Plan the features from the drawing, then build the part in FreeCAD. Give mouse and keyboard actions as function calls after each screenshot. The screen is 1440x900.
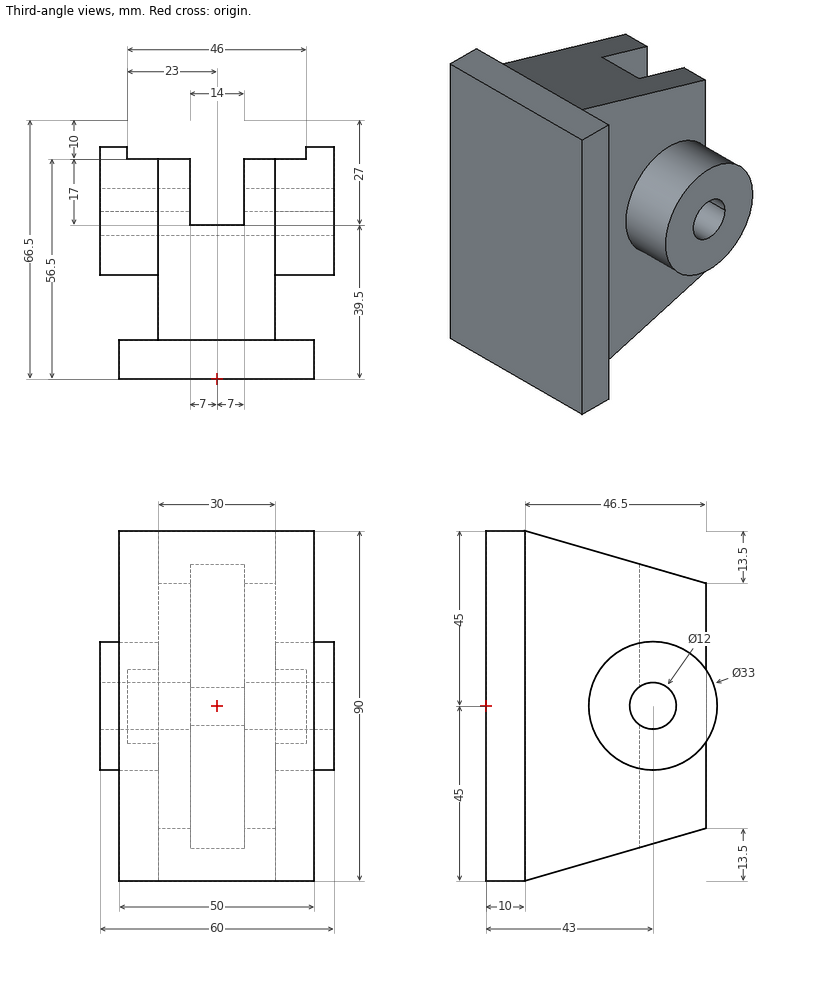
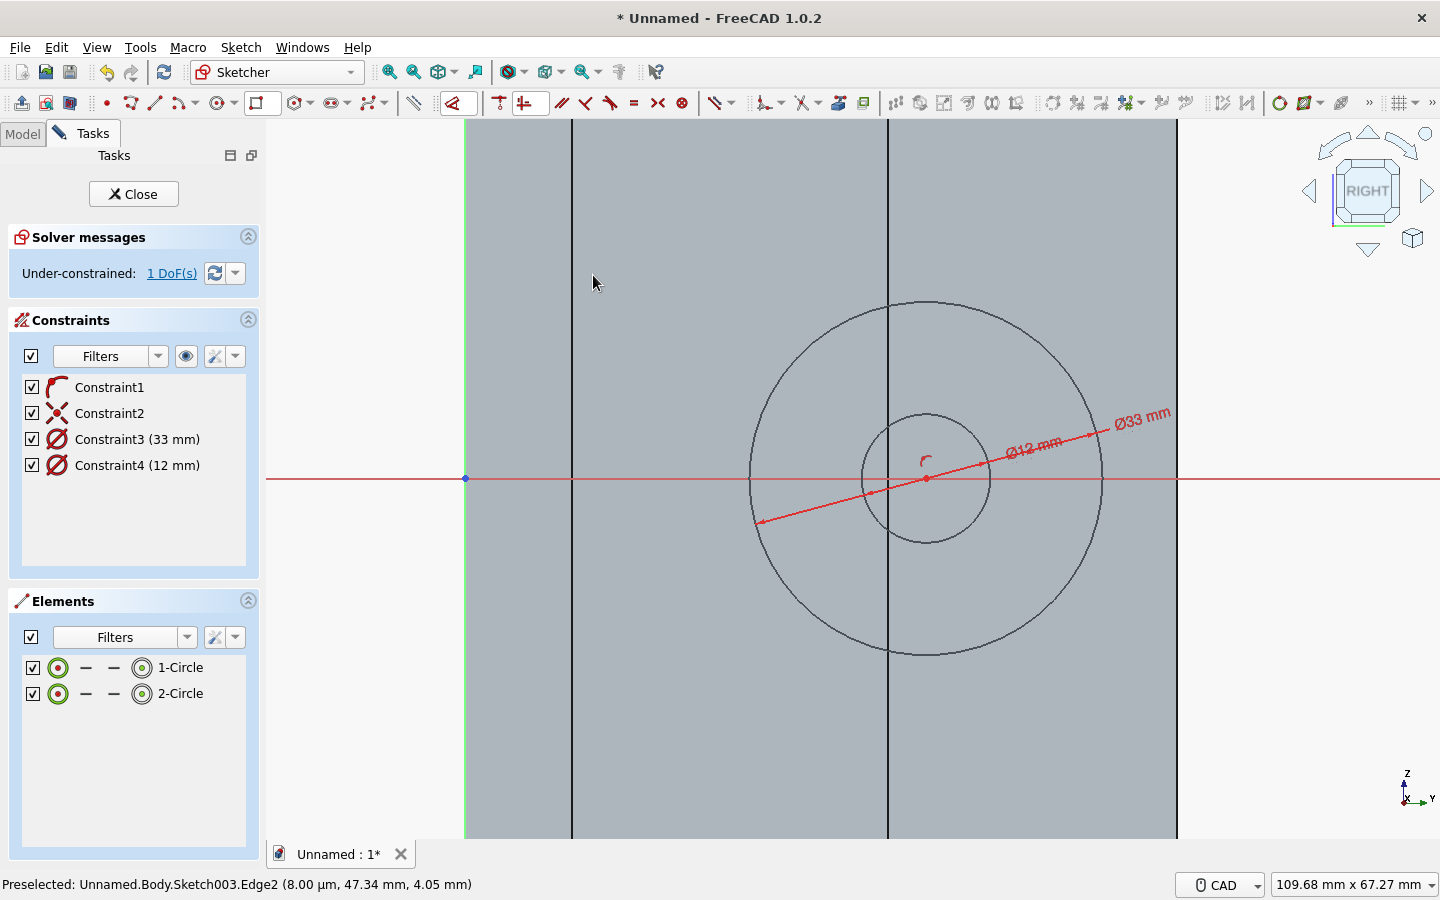
click(926, 479)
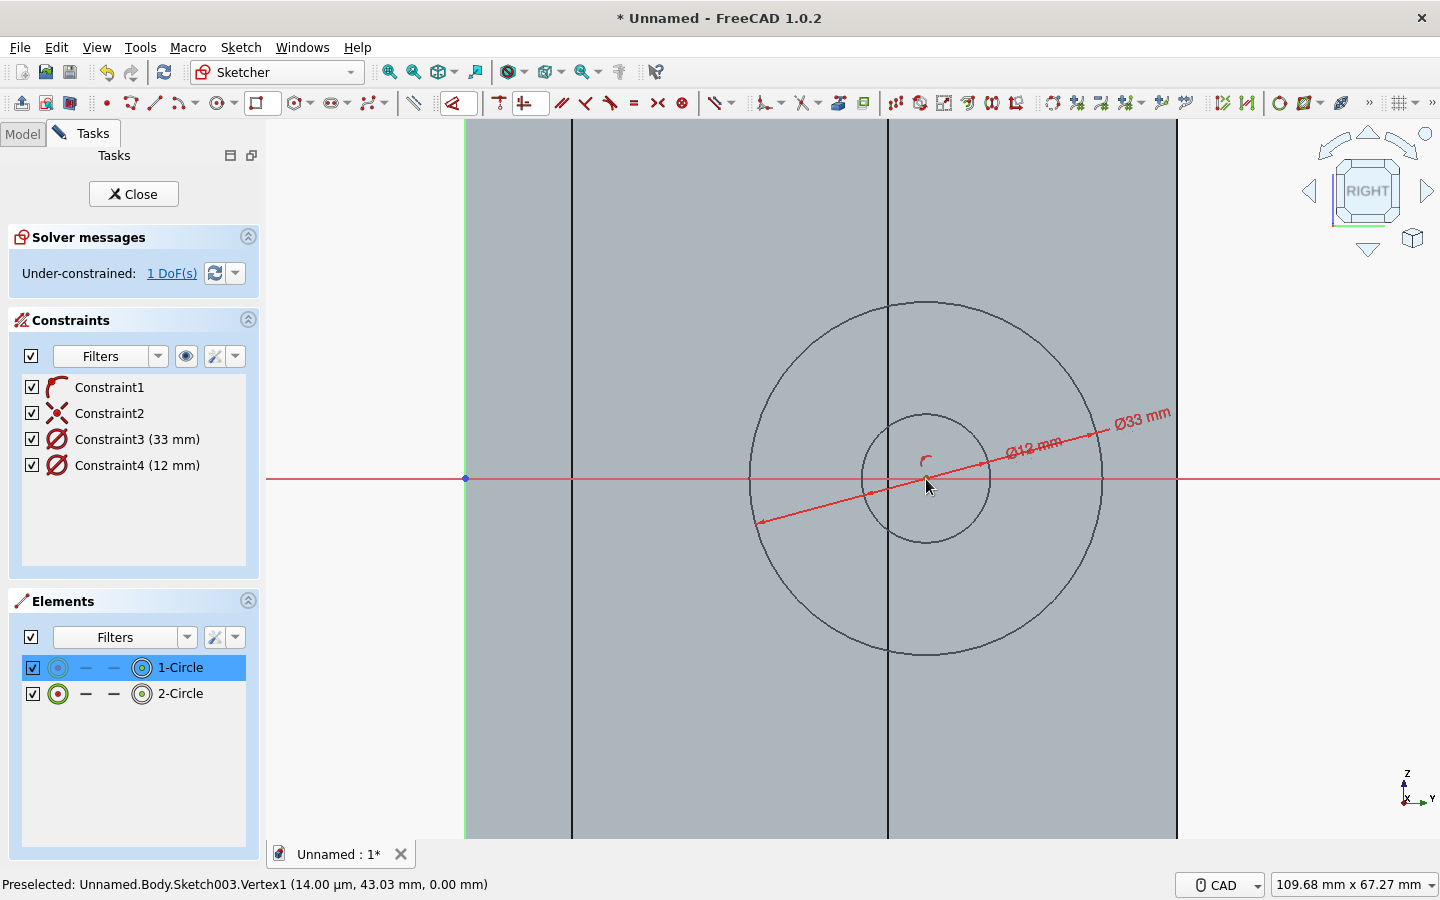
click(472, 104)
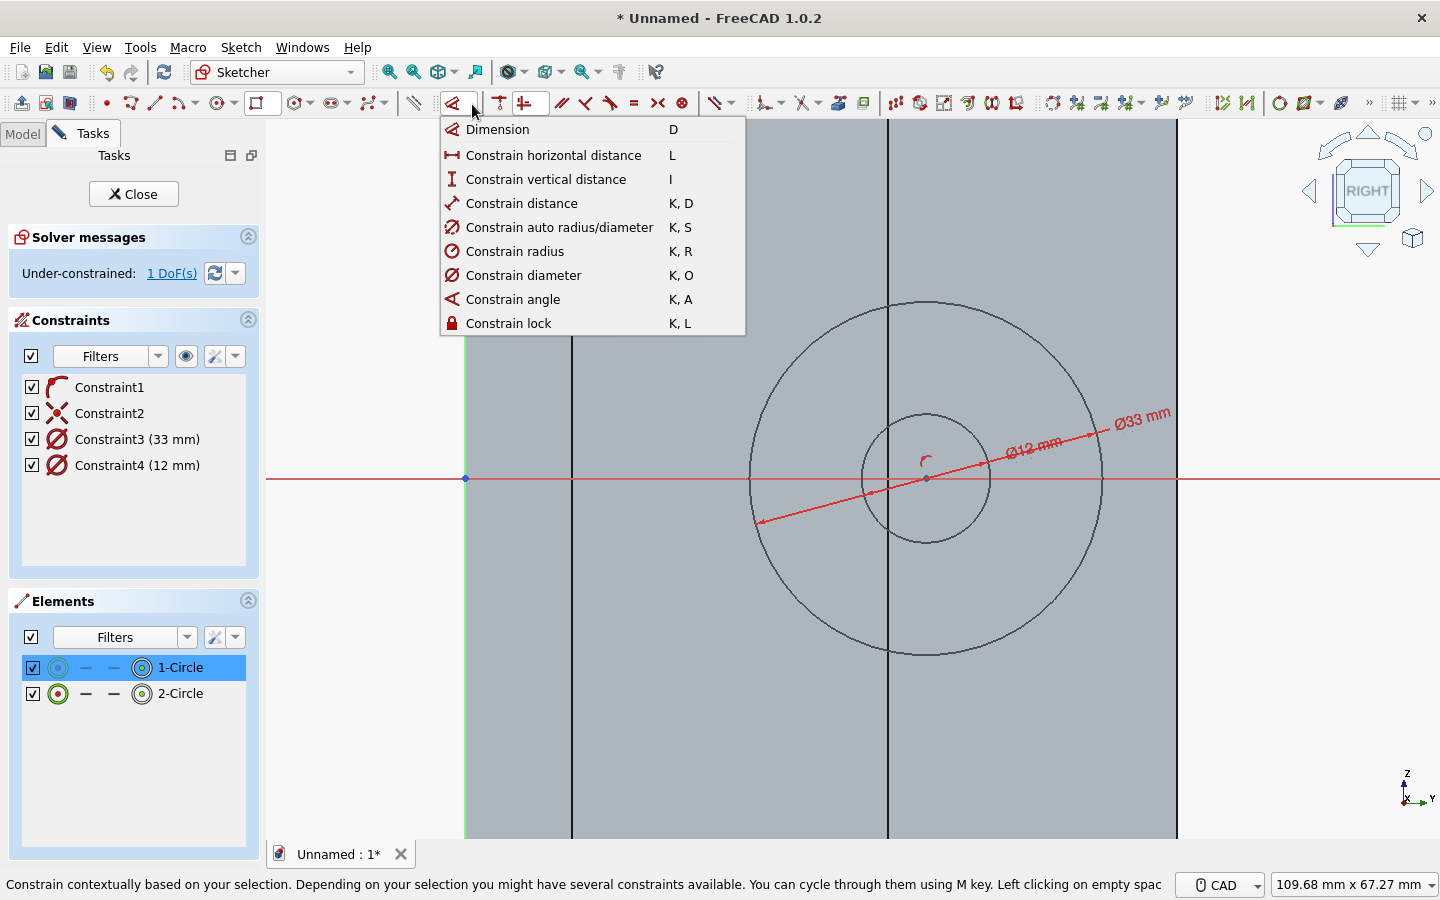
click(593, 155)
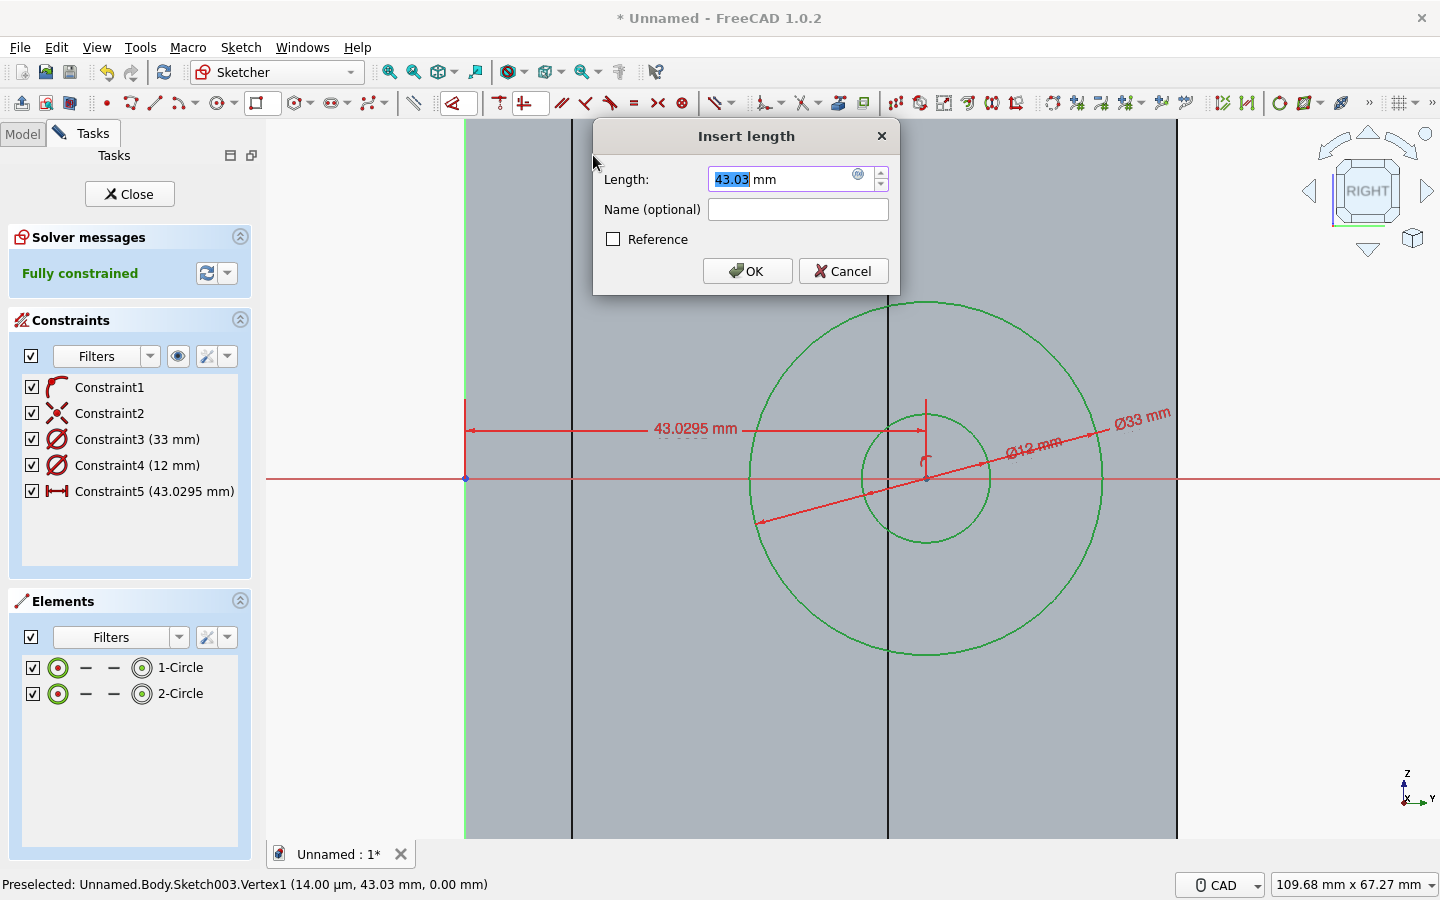
text(43)
key(Return)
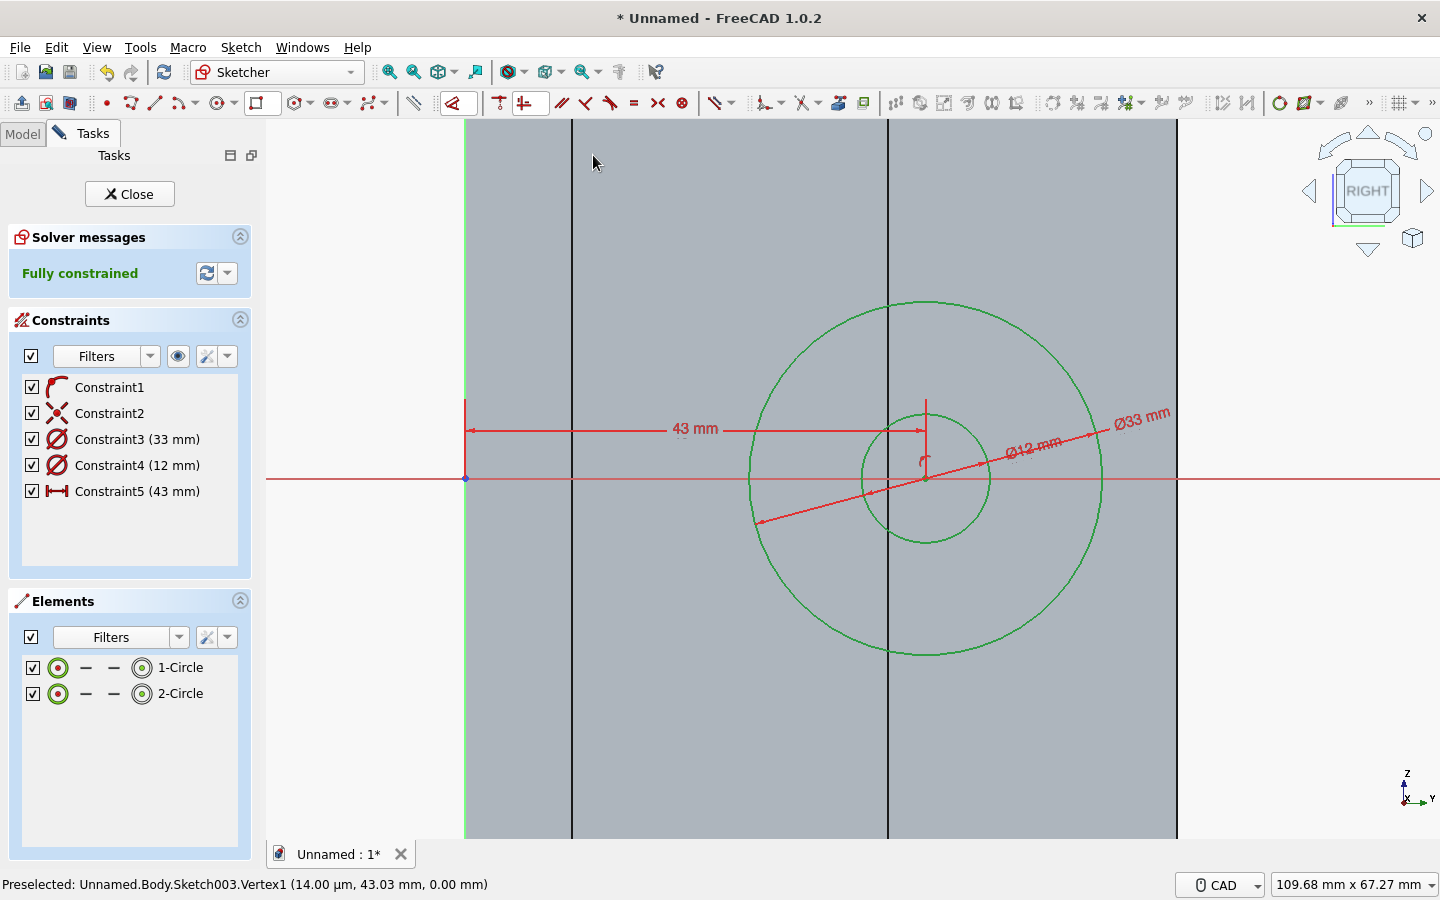
click(130, 194)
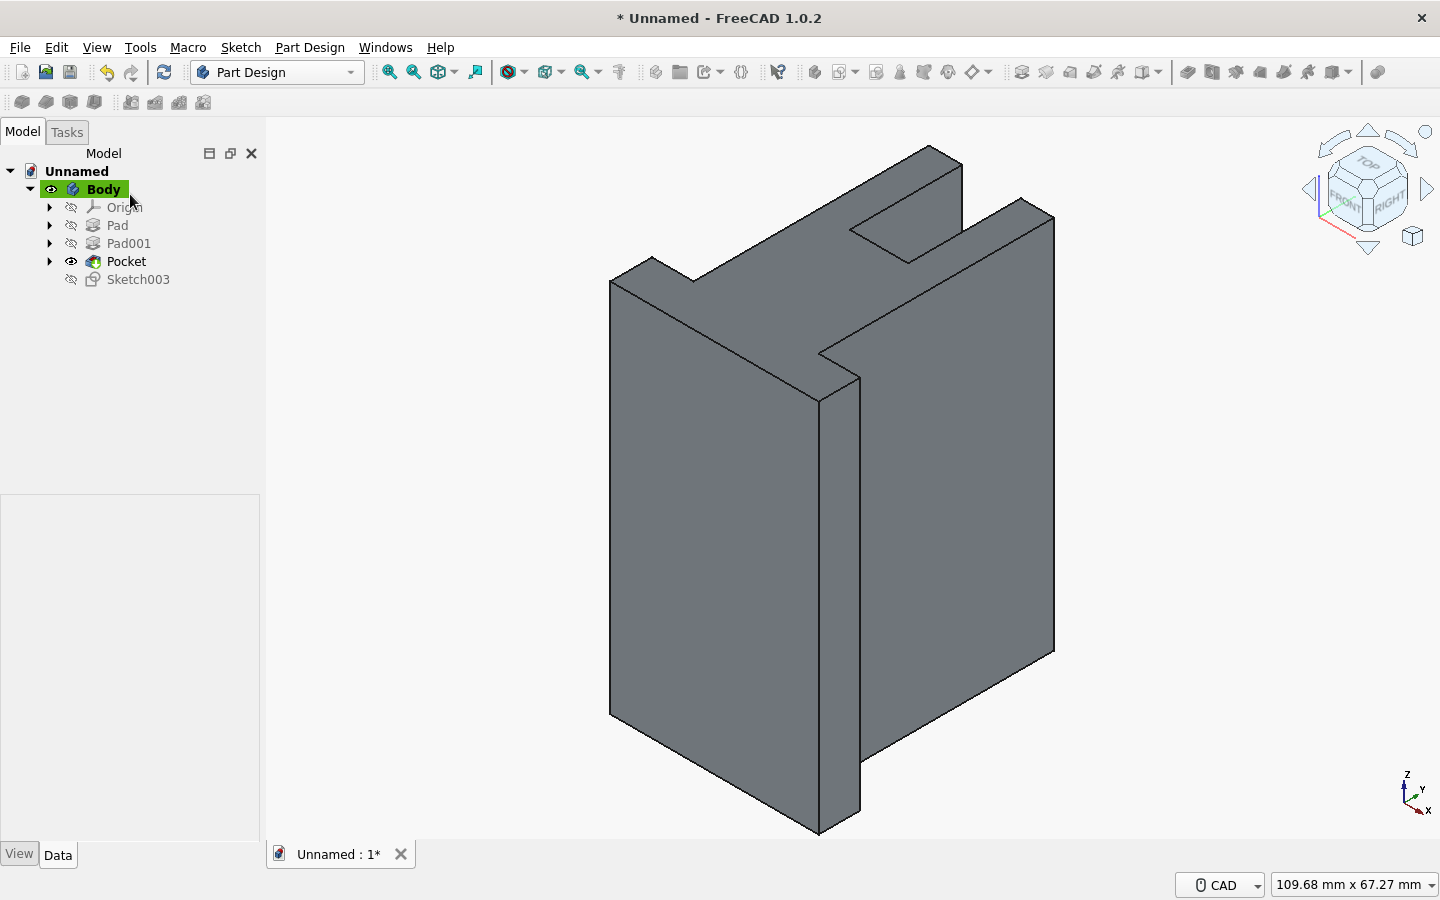
click(1022, 72)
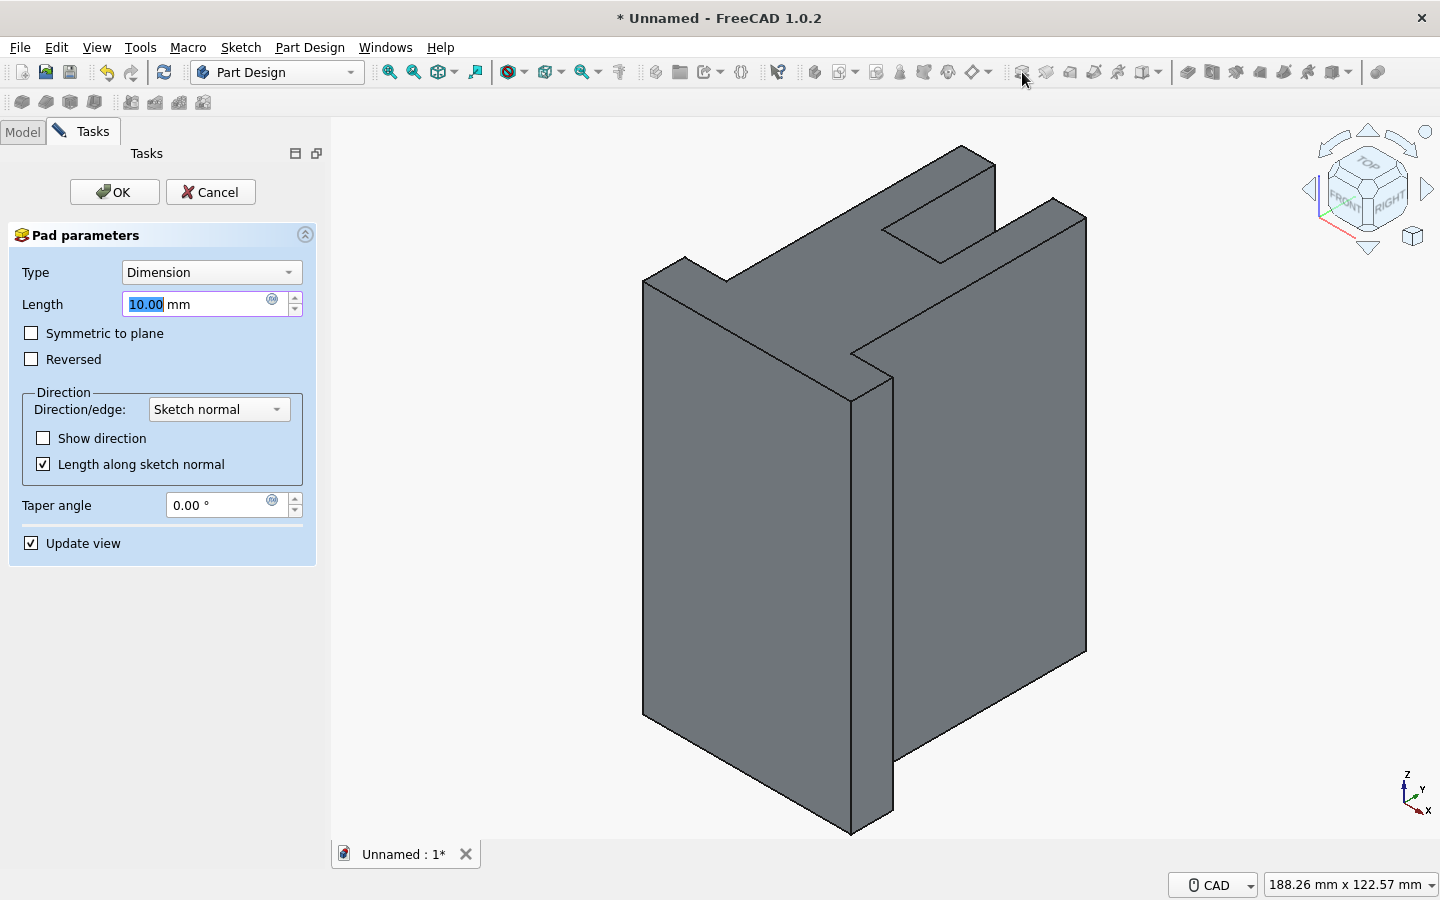
text(60)
key(Tab)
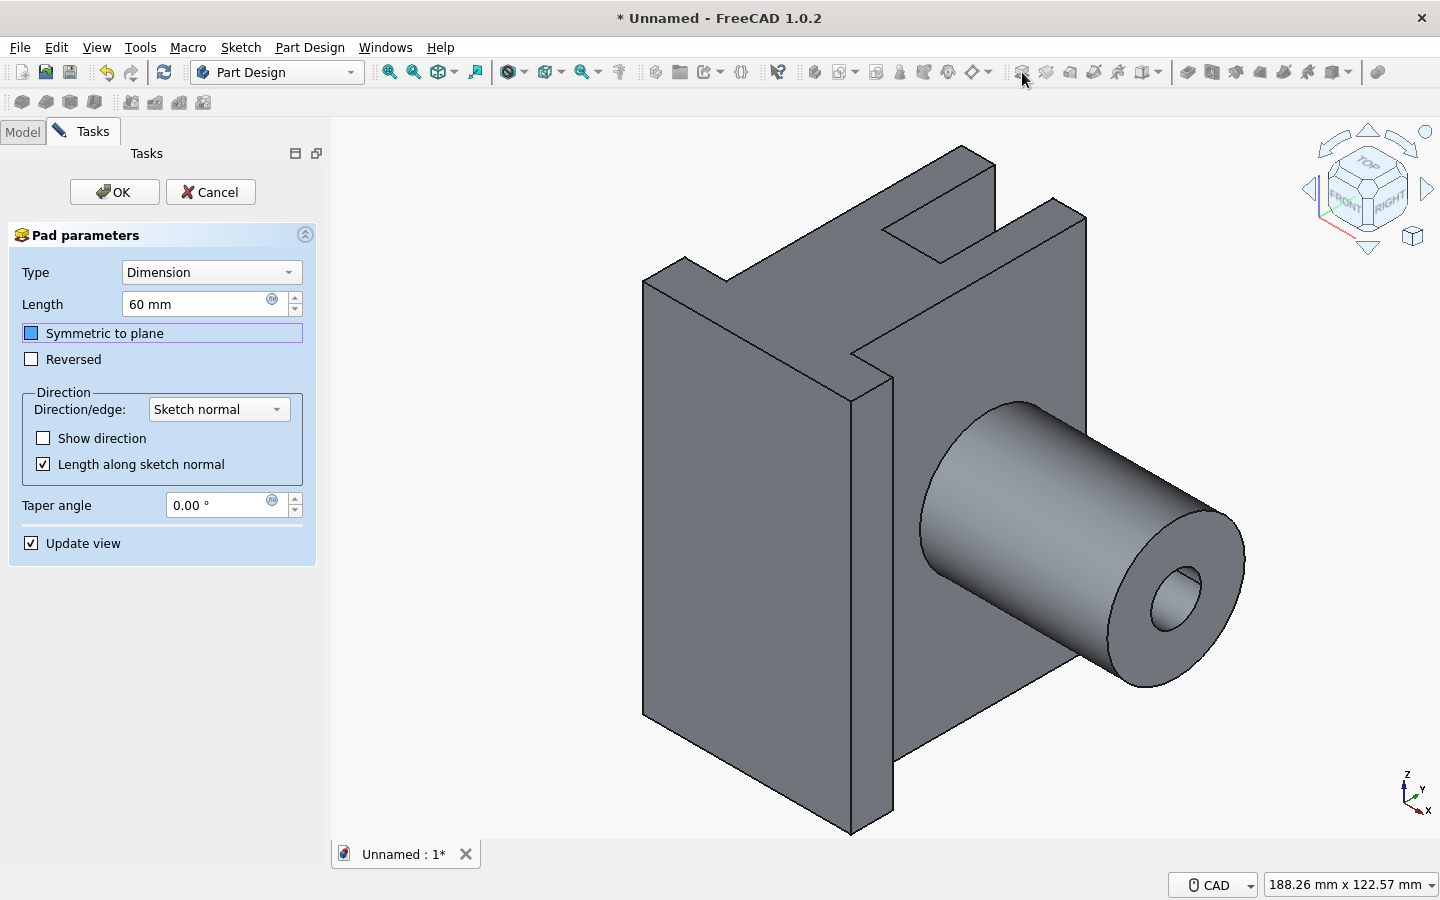
click(30, 333)